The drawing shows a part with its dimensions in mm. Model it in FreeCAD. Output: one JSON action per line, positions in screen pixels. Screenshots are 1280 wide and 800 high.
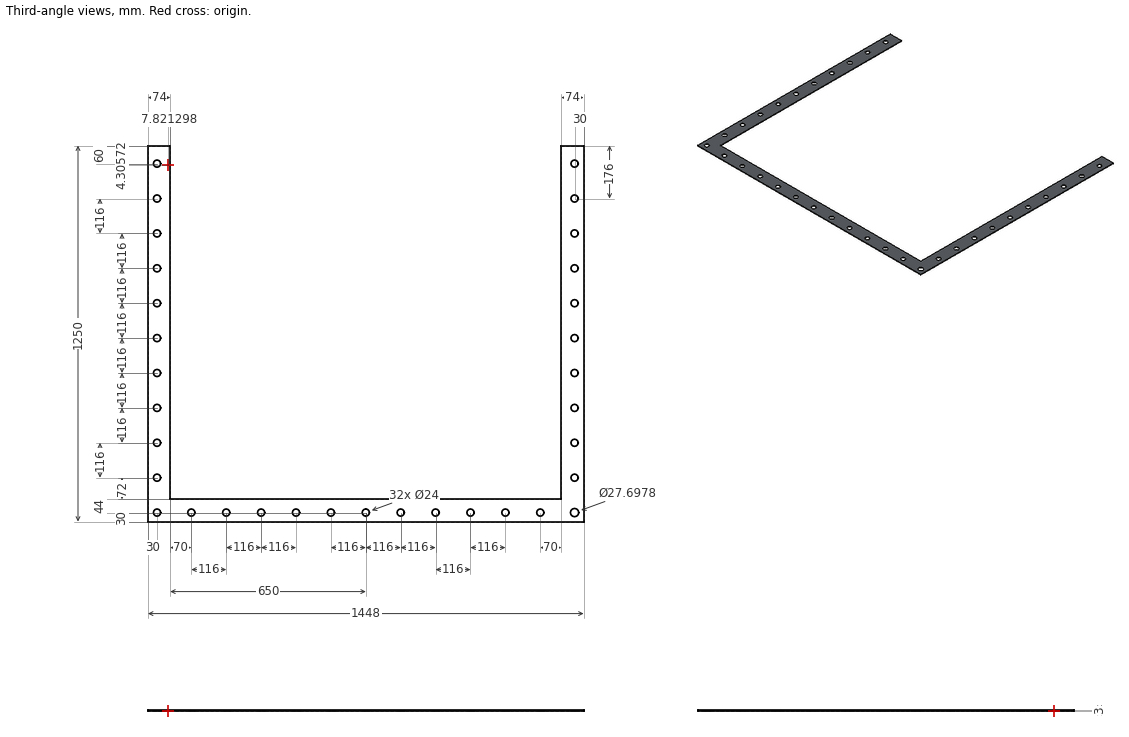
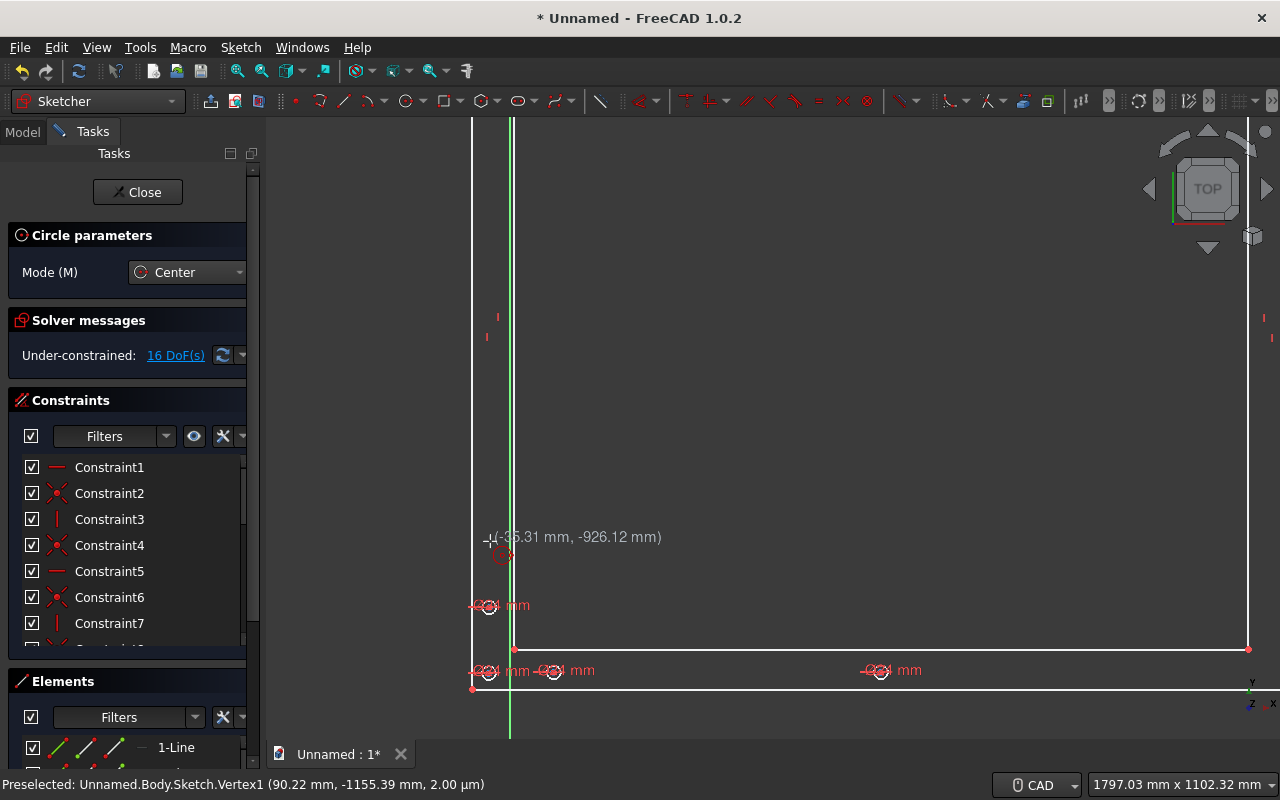
{"action": "left_click", "coordinate": [489, 541]}
{"action": "mouse_move", "coordinate": [494, 536]}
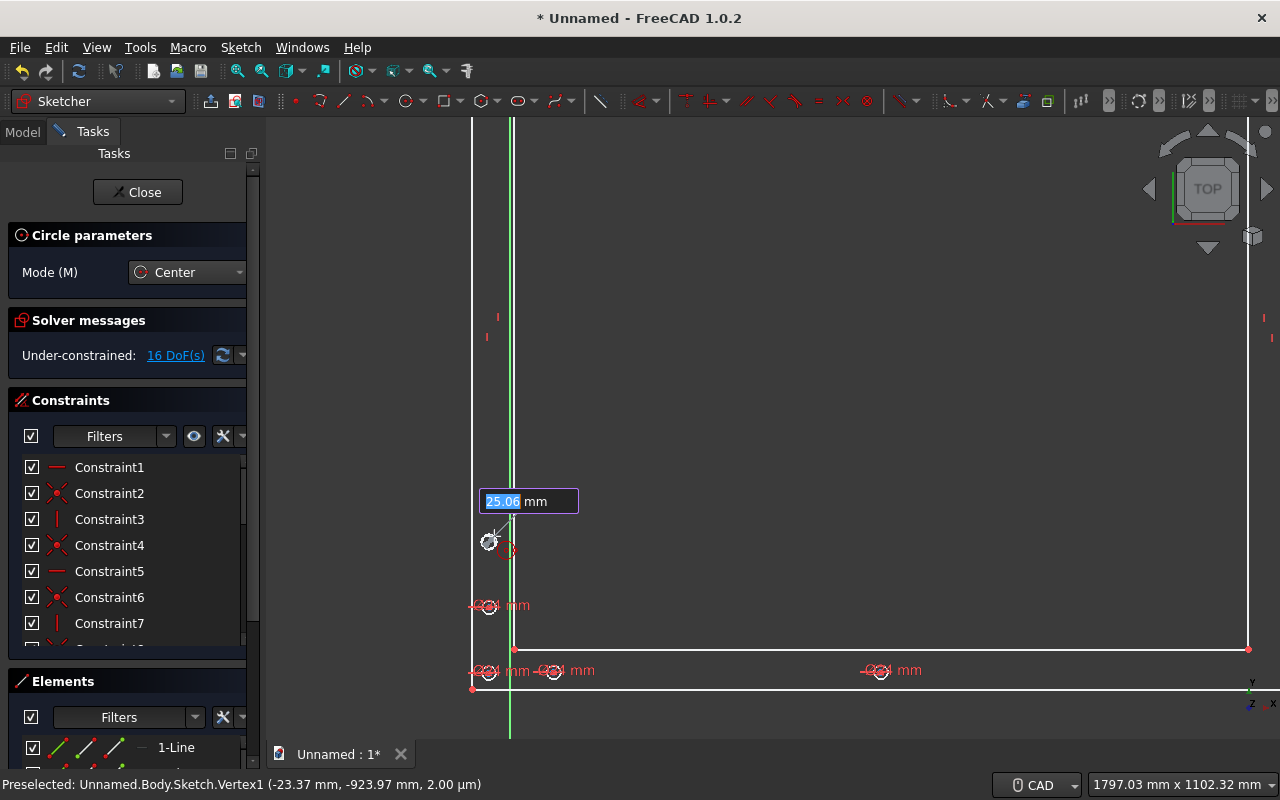
{"action": "type", "text": "24"}
{"action": "key", "text": "Return"}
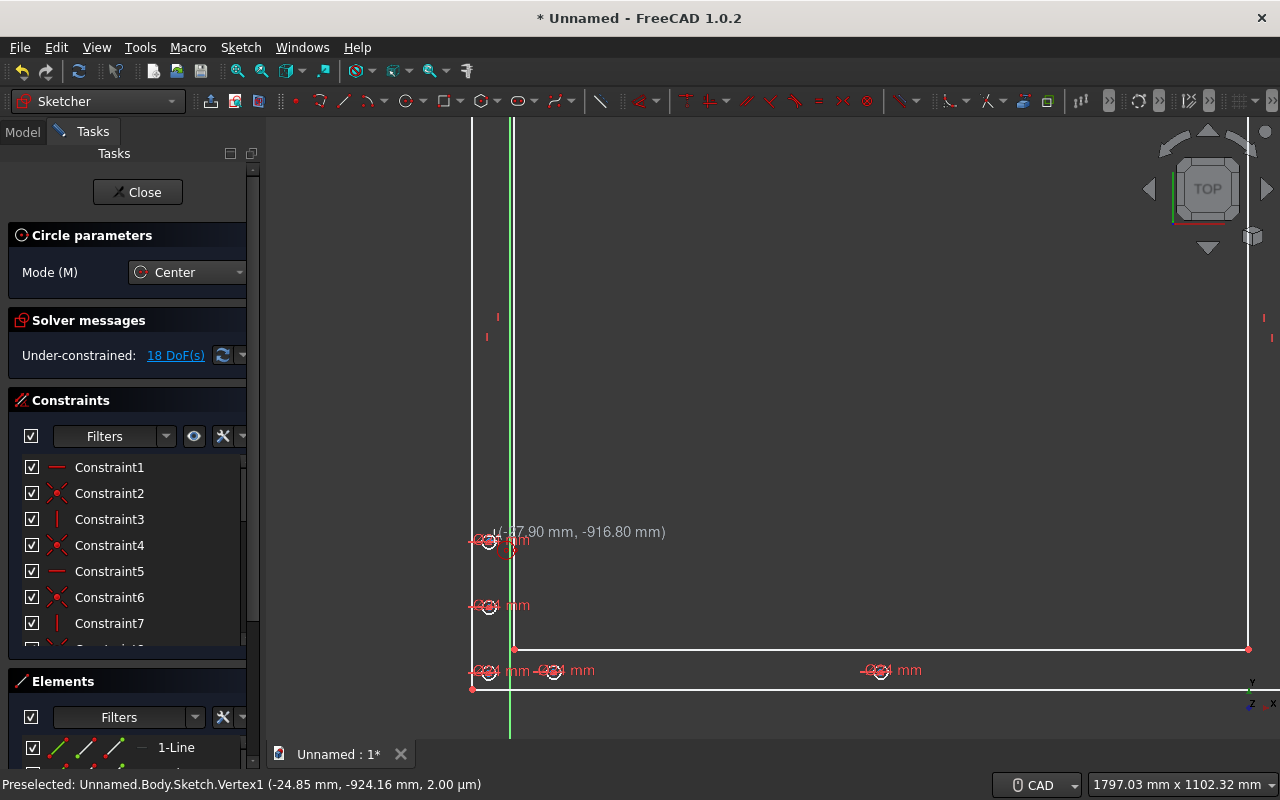
{"action": "scroll", "coordinate": [619, 672], "scroll_direction": "up", "scroll_amount": 7}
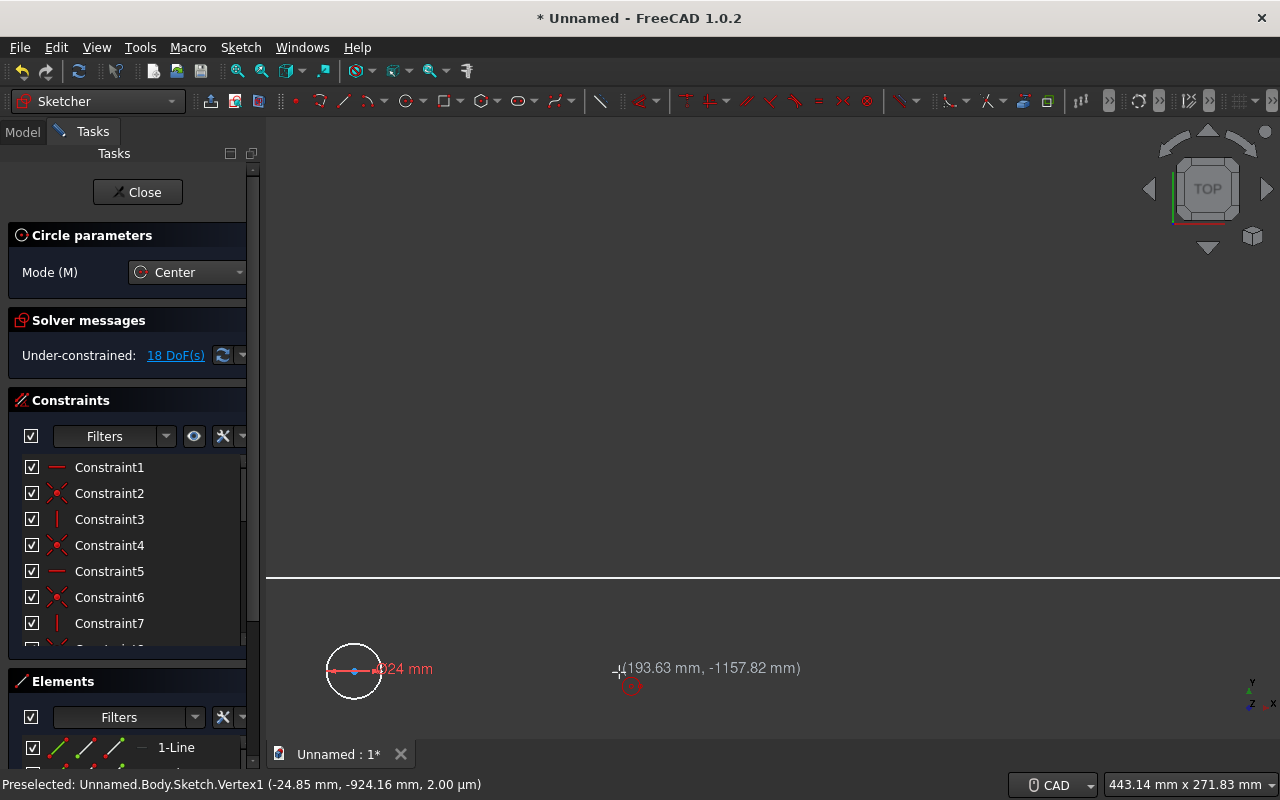
{"action": "scroll", "coordinate": [552, 603], "scroll_direction": "down", "scroll_amount": 10}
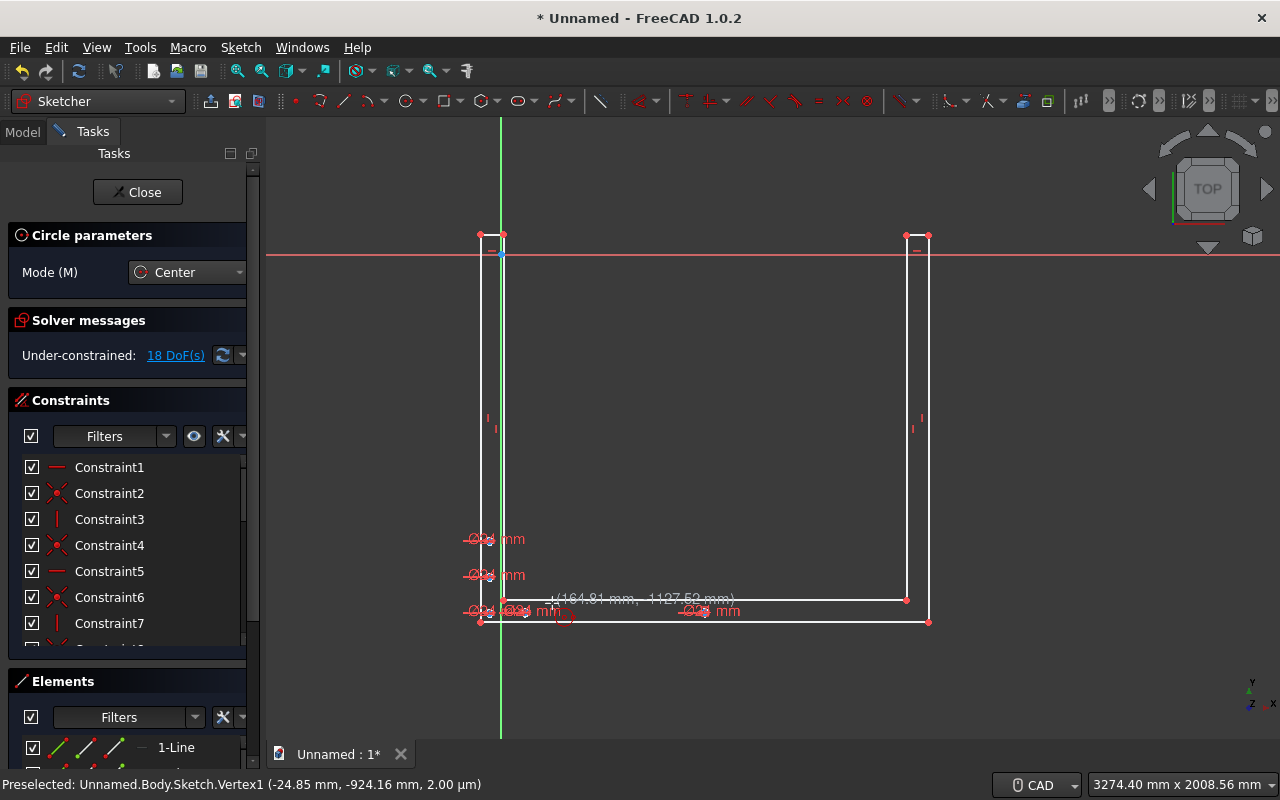
{"action": "scroll", "coordinate": [561, 613], "scroll_direction": "up", "scroll_amount": 3}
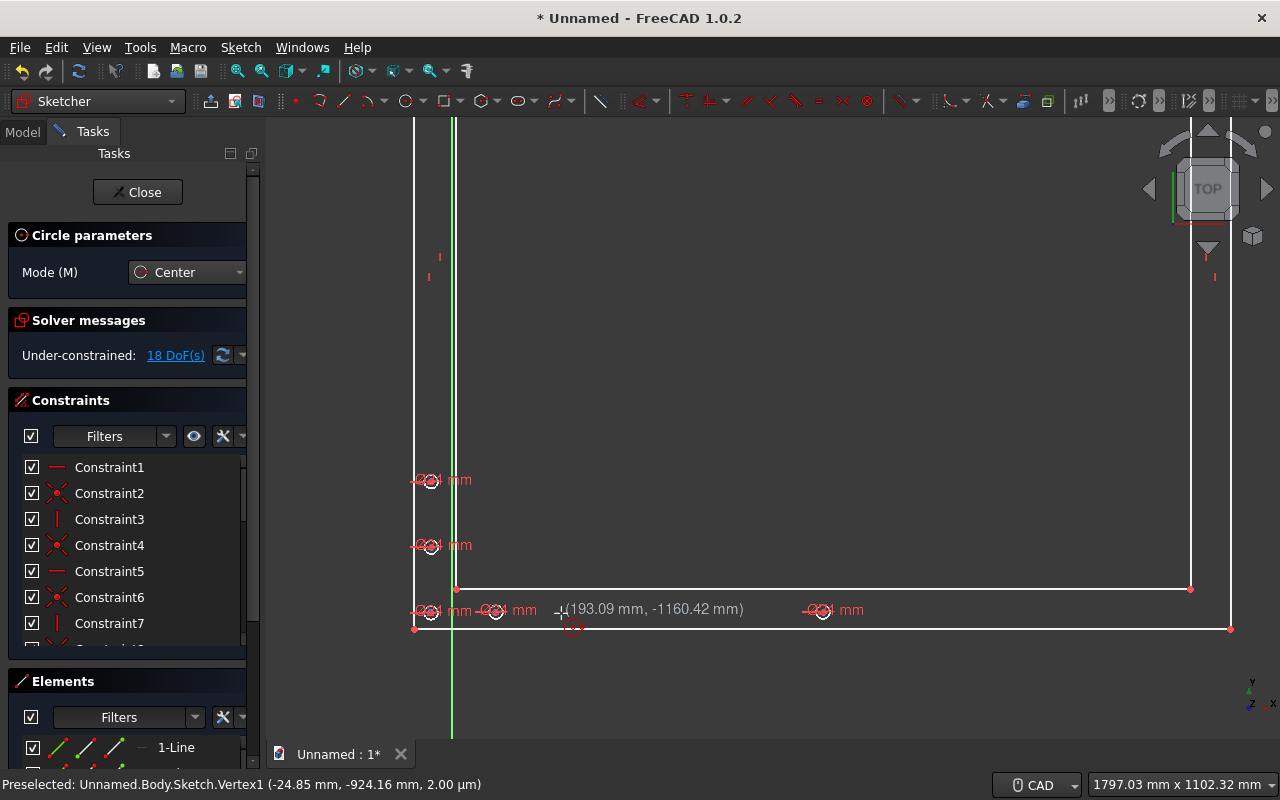
{"action": "left_click", "coordinate": [561, 611]}
{"action": "mouse_move", "coordinate": [566, 607]}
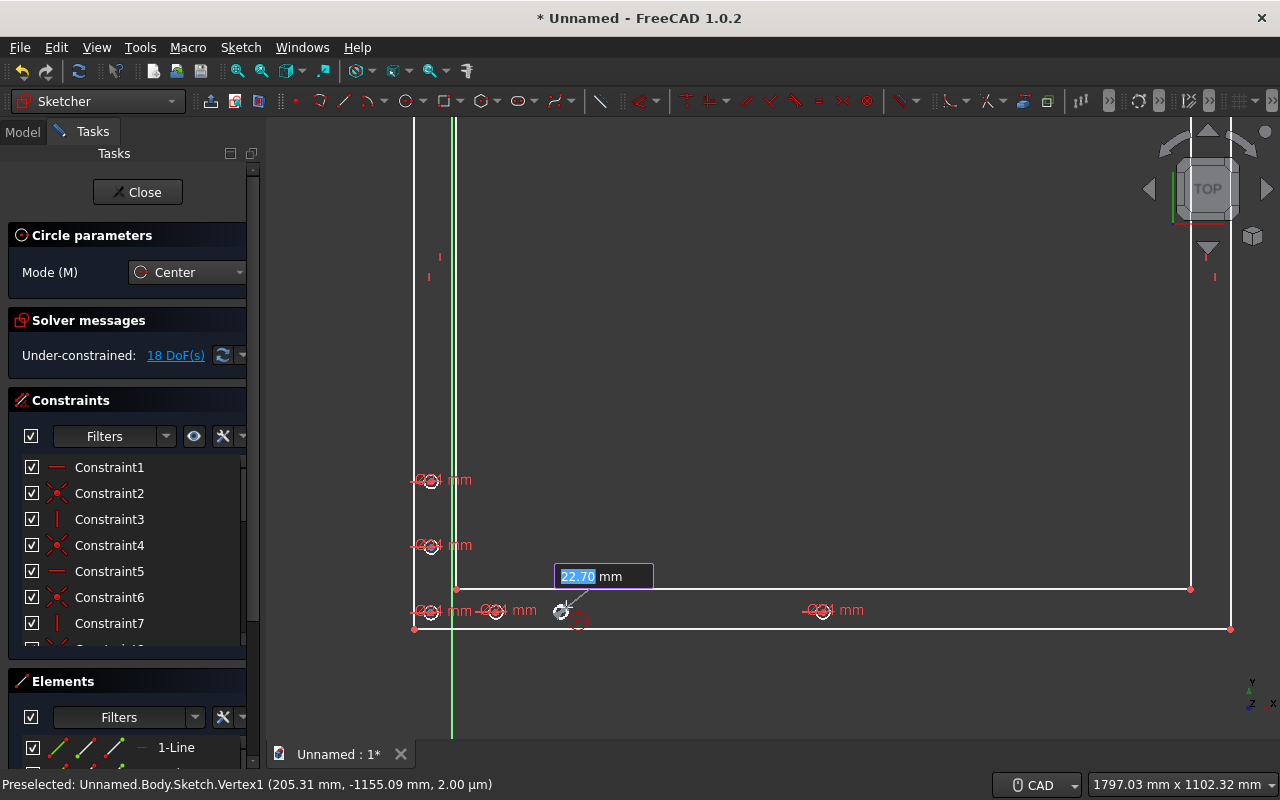
{"action": "type", "text": "24"}
{"action": "key", "text": "Return"}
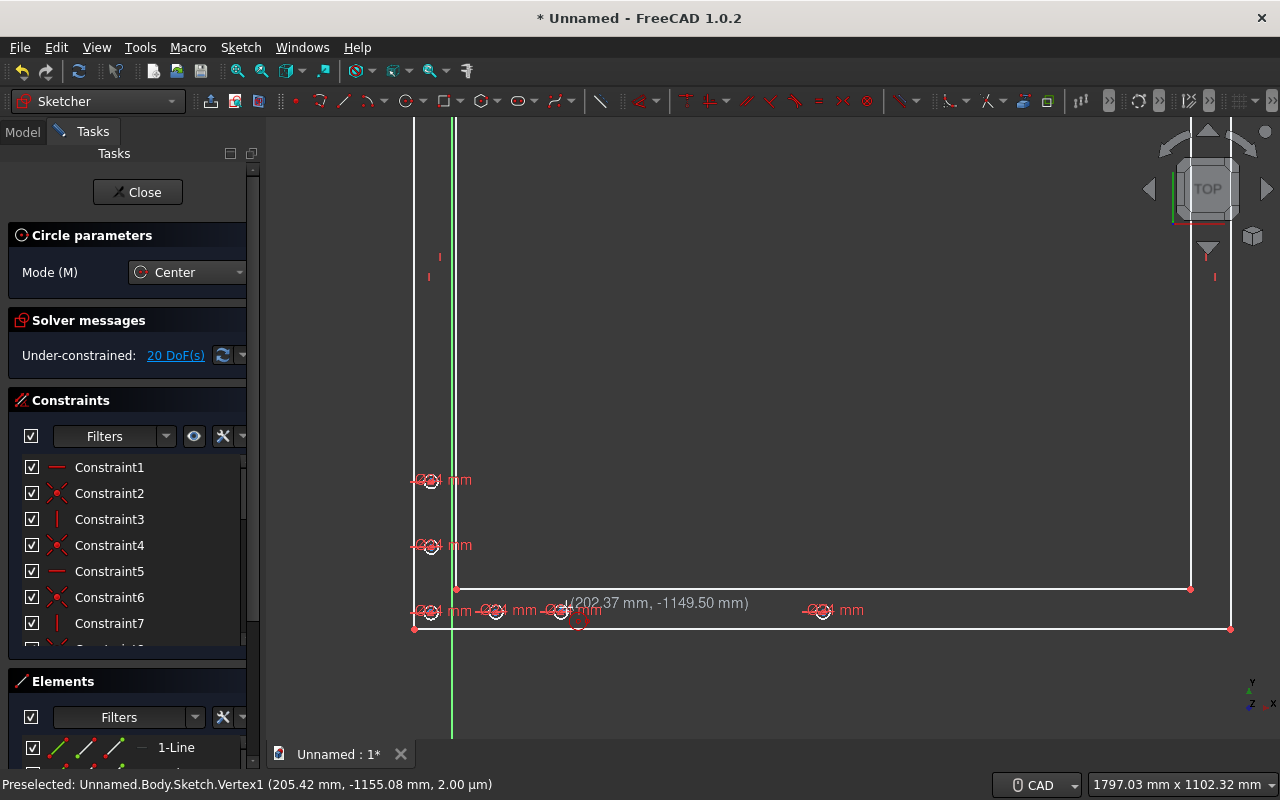
{"action": "scroll", "coordinate": [431, 415], "scroll_direction": "up", "scroll_amount": 7}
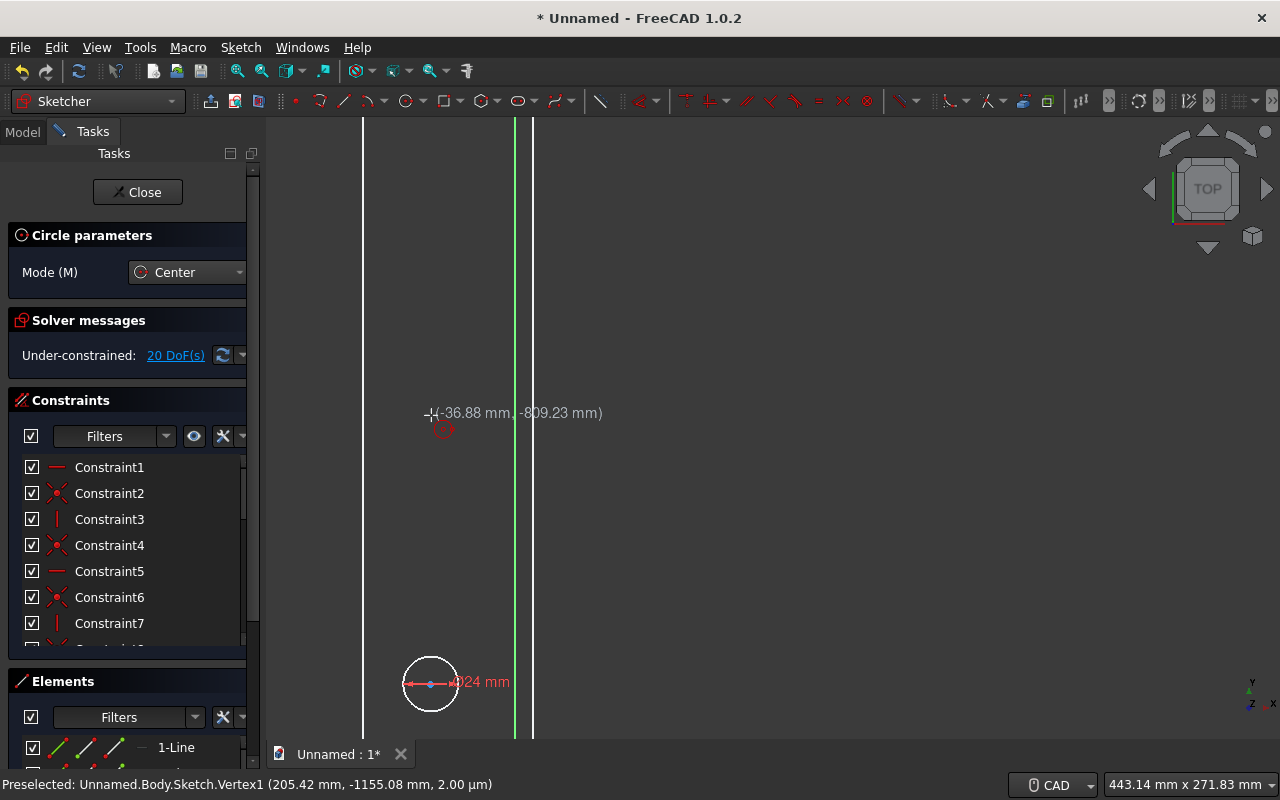
{"action": "scroll", "coordinate": [499, 519], "scroll_direction": "down", "scroll_amount": 10}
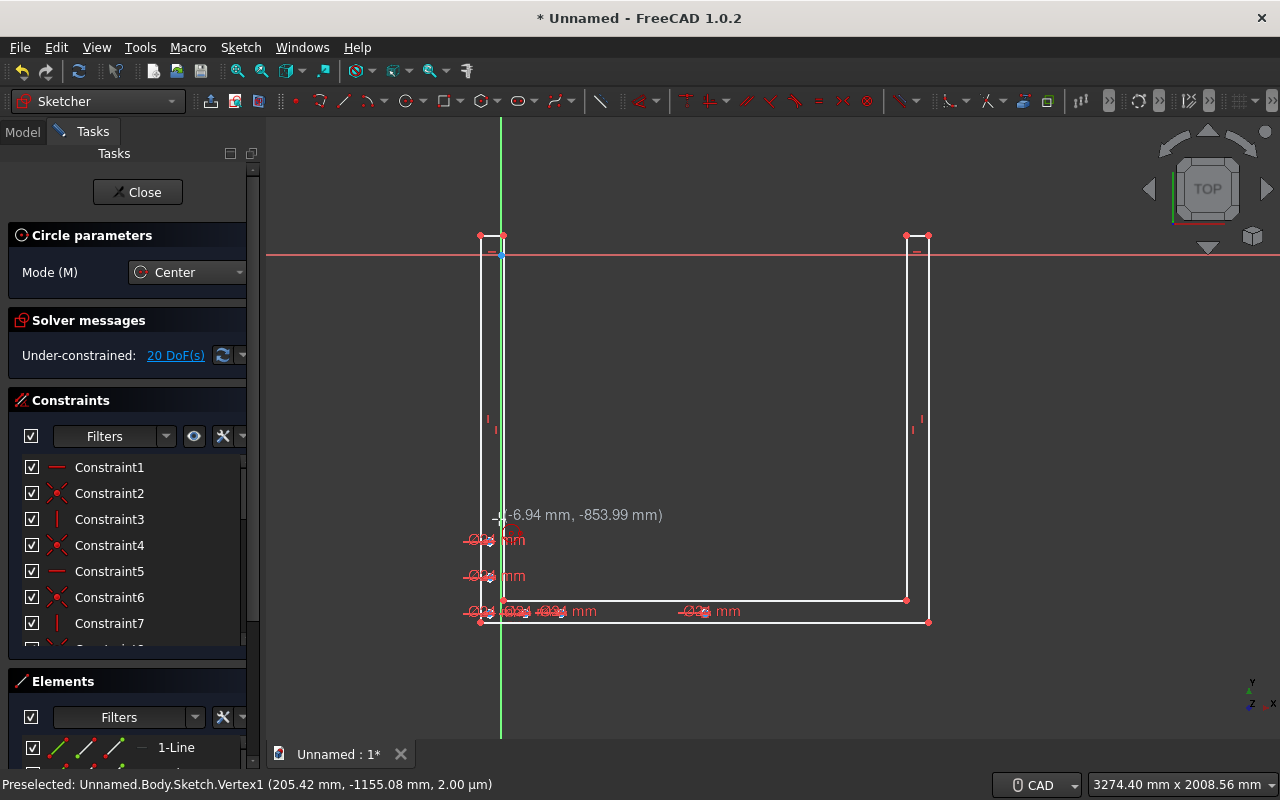
{"action": "scroll", "coordinate": [490, 505], "scroll_direction": "up", "scroll_amount": 3}